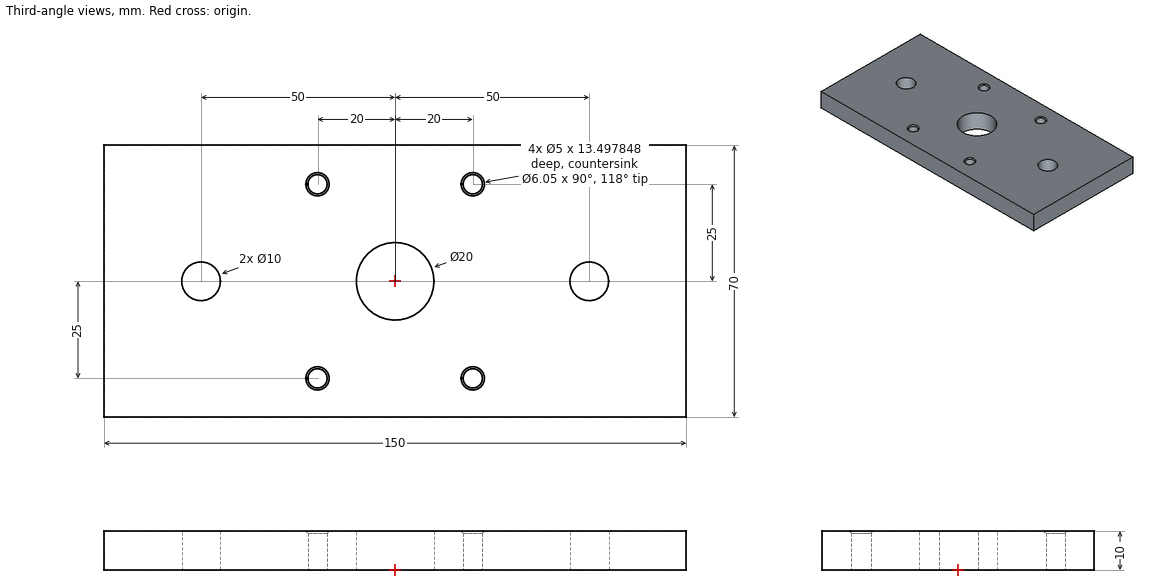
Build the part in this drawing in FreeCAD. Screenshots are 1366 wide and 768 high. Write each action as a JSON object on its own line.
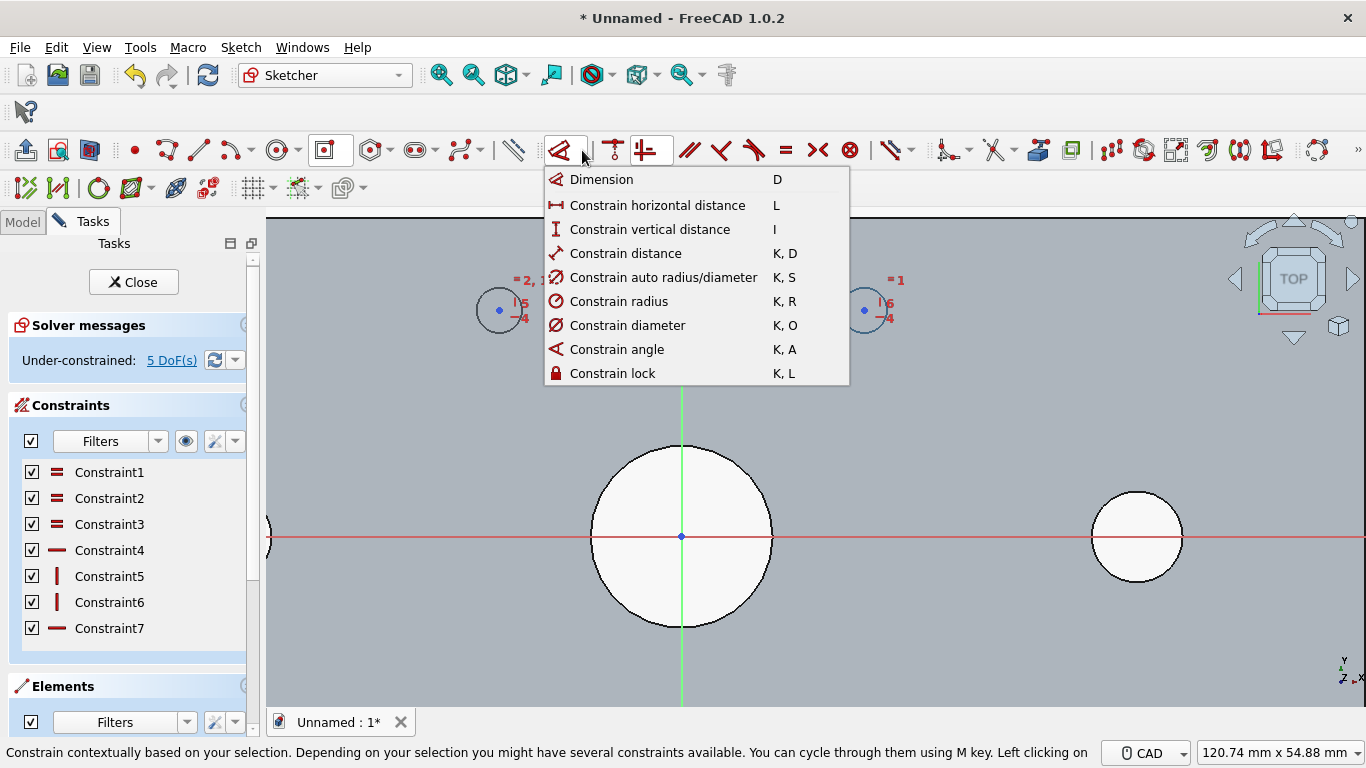
{"action": "left_click", "coordinate": [697, 325]}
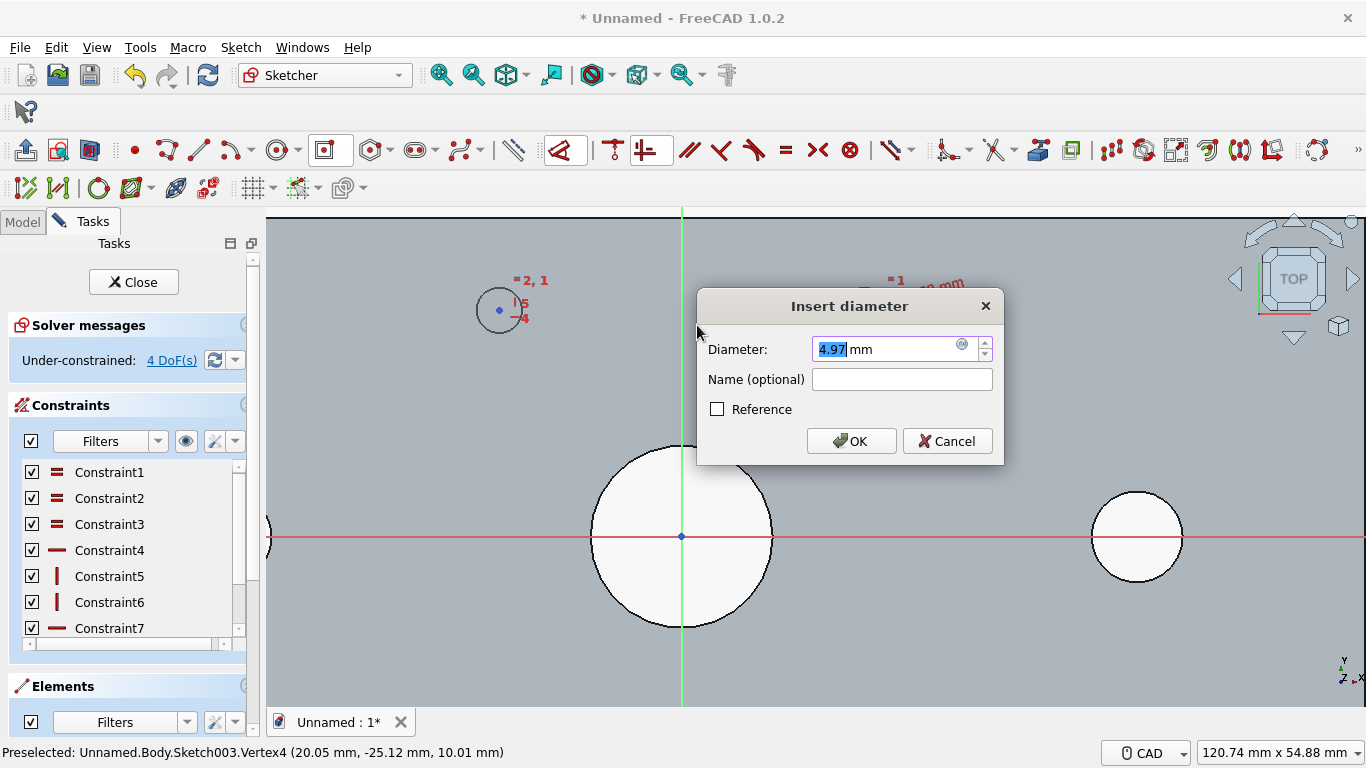
{"action": "type", "text": "5"}
{"action": "key", "text": "Return"}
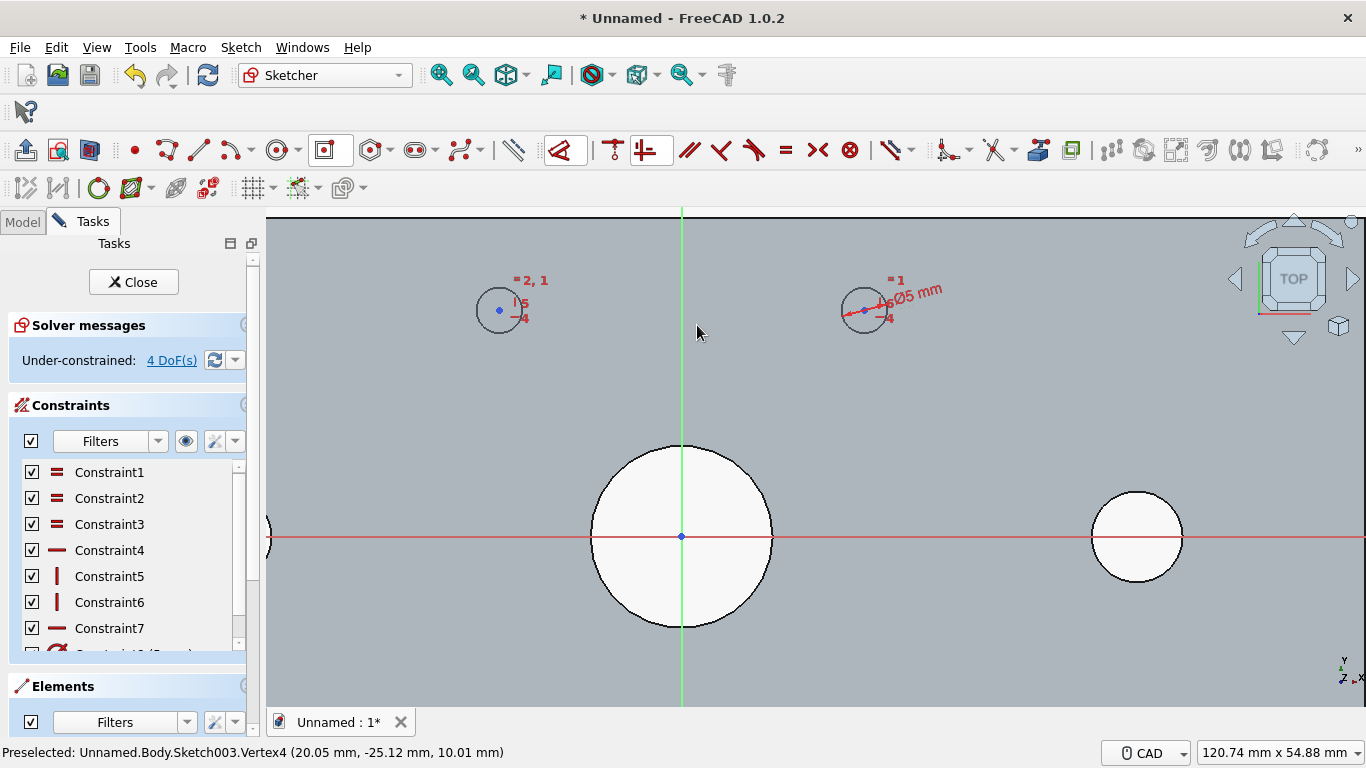
{"action": "left_click", "coordinate": [864, 310]}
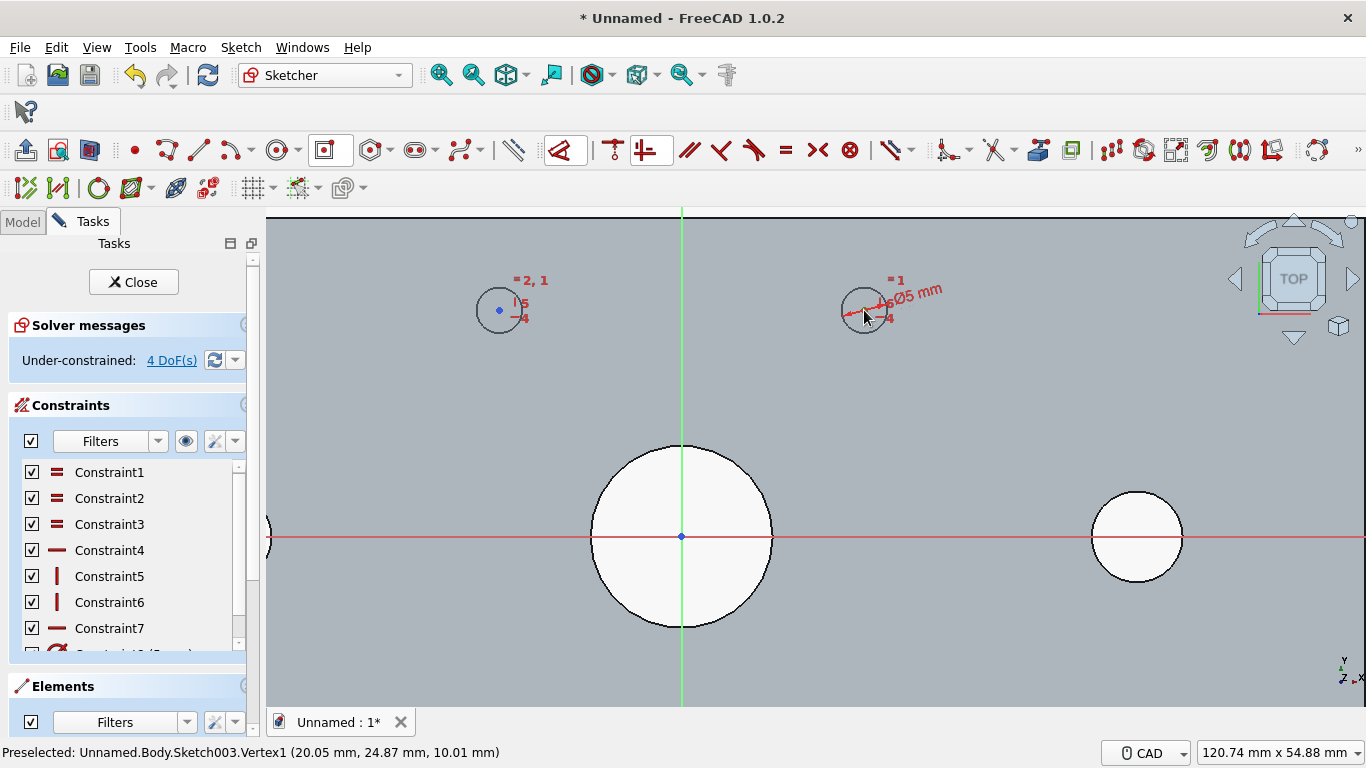
{"action": "key", "text": "l"}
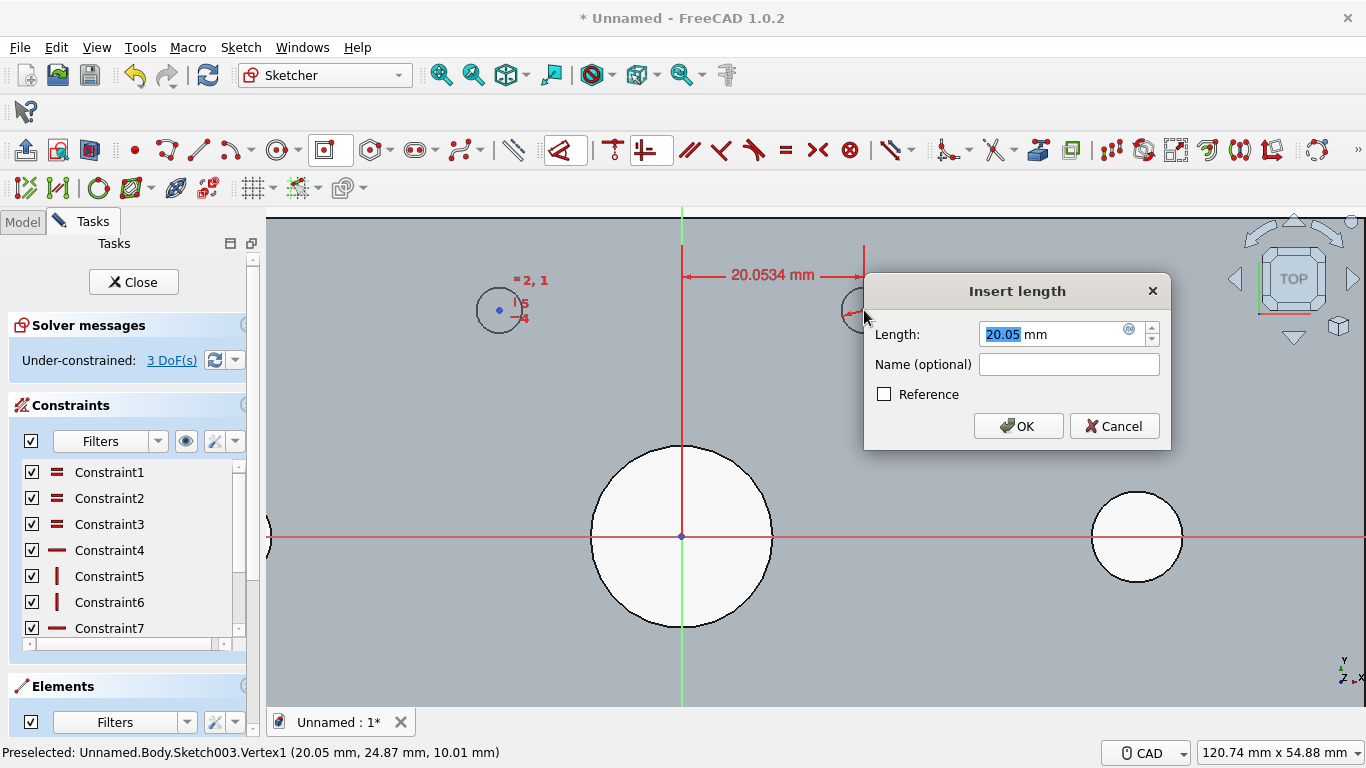
{"action": "type", "text": "20"}
{"action": "key", "text": "Return"}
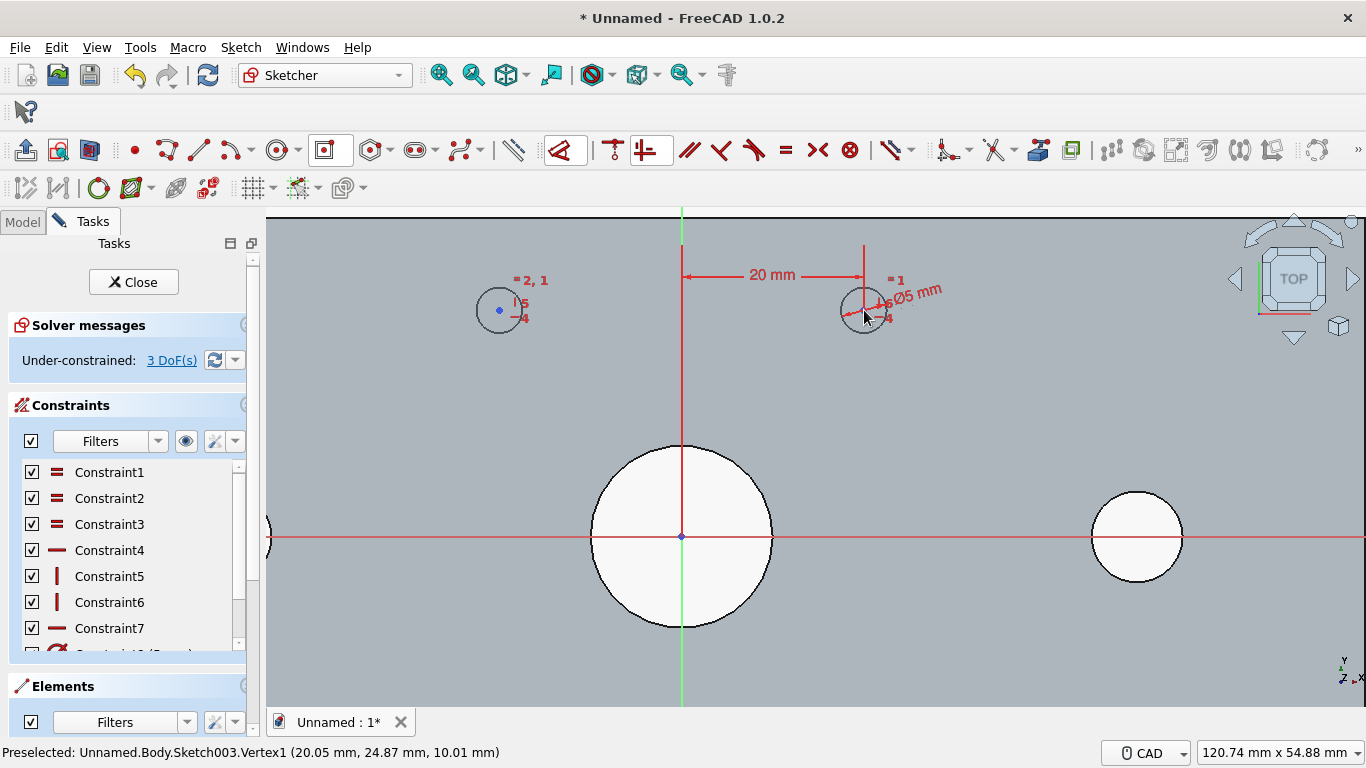
{"action": "left_click", "coordinate": [864, 310]}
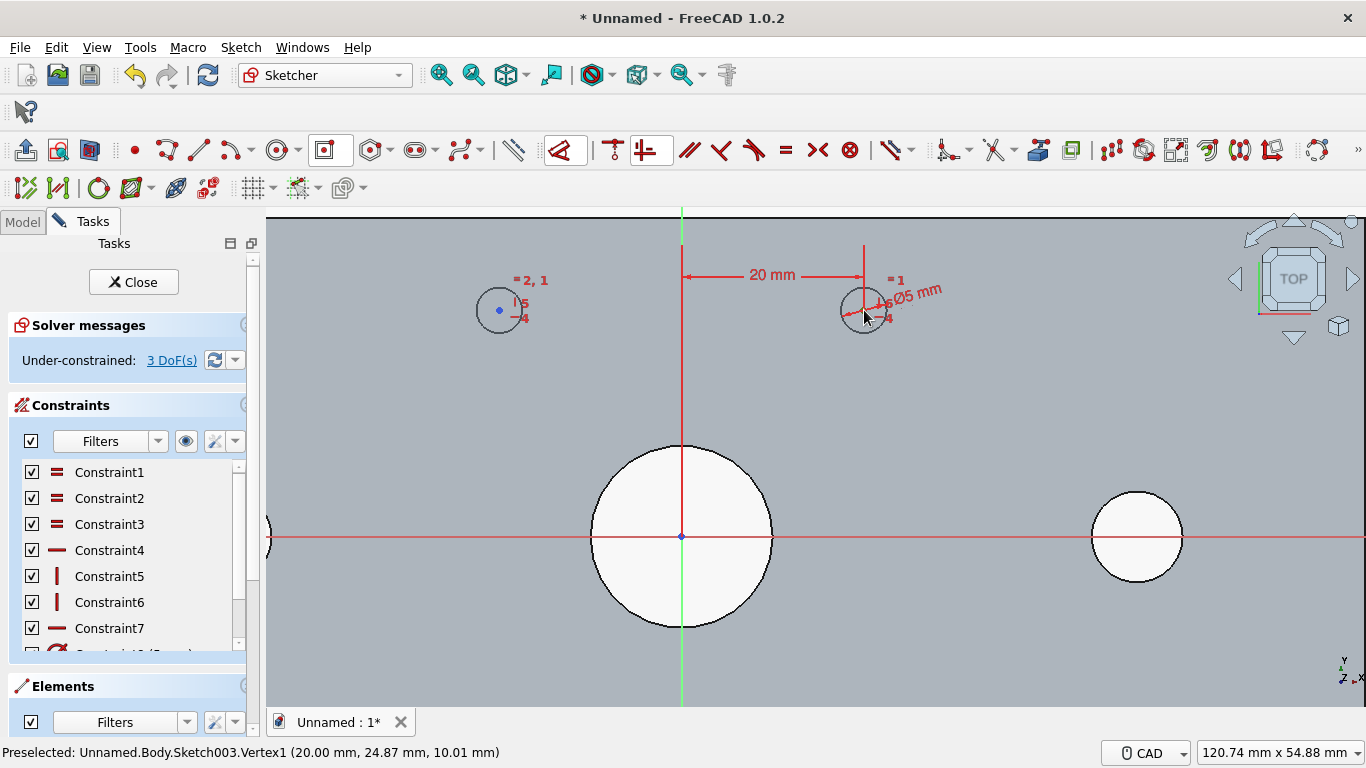
{"action": "key", "text": "i"}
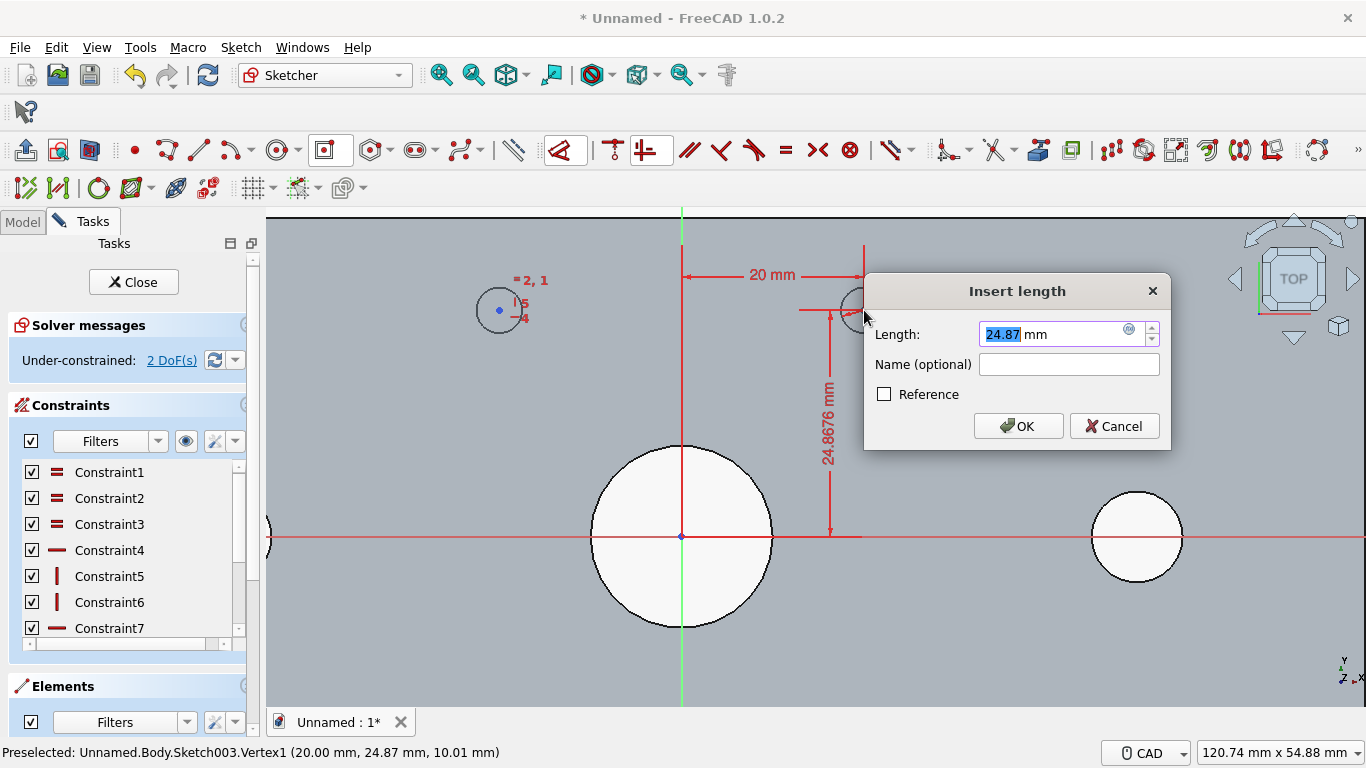
{"action": "type", "text": "25"}
{"action": "key", "text": "Return"}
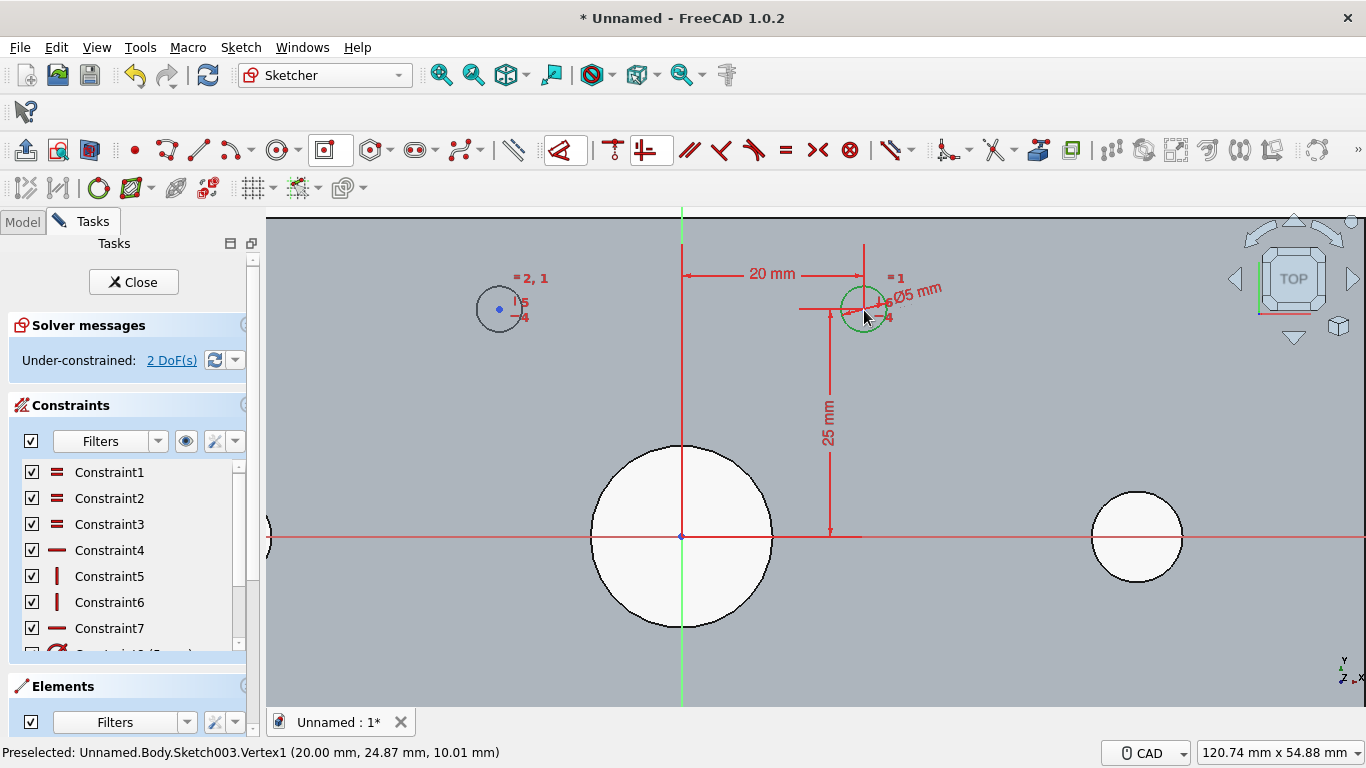
{"action": "left_click", "coordinate": [499, 309]}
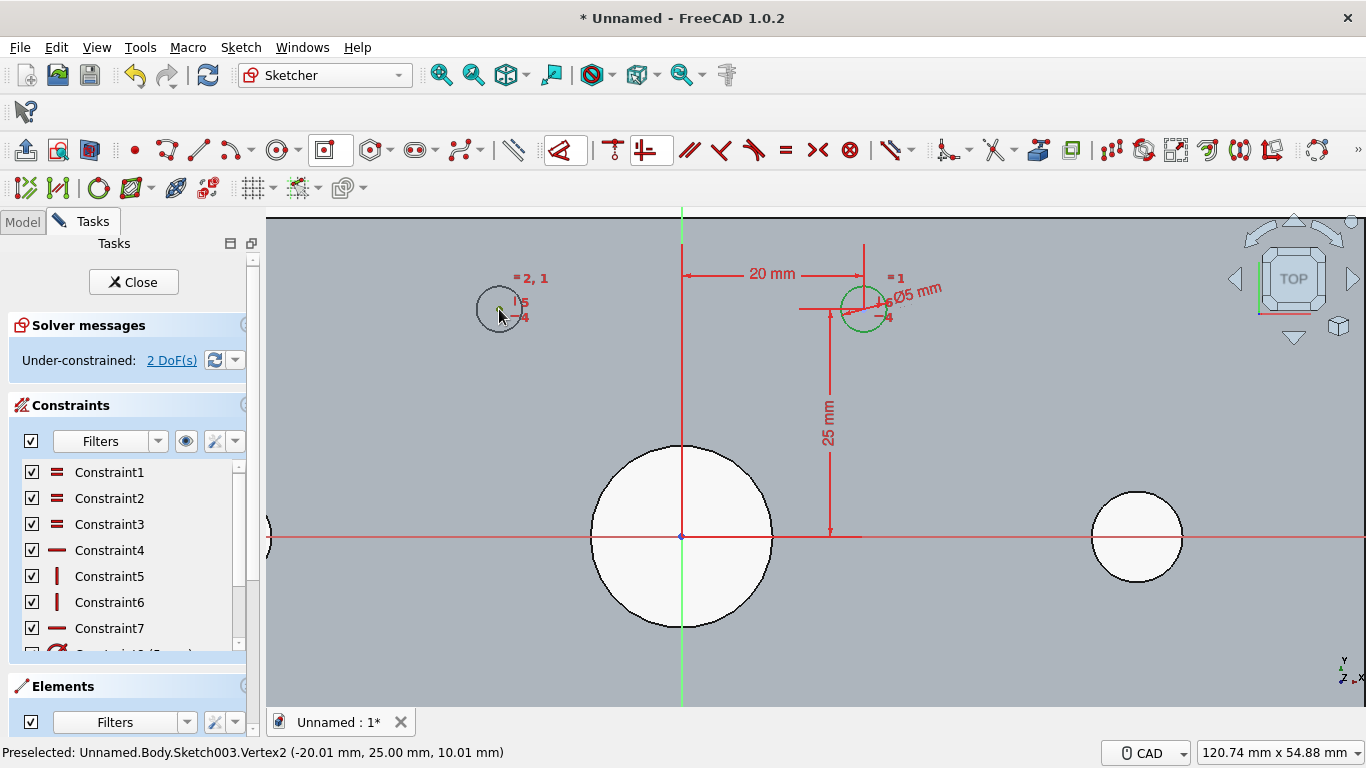
{"action": "left_click", "coordinate": [582, 150]}